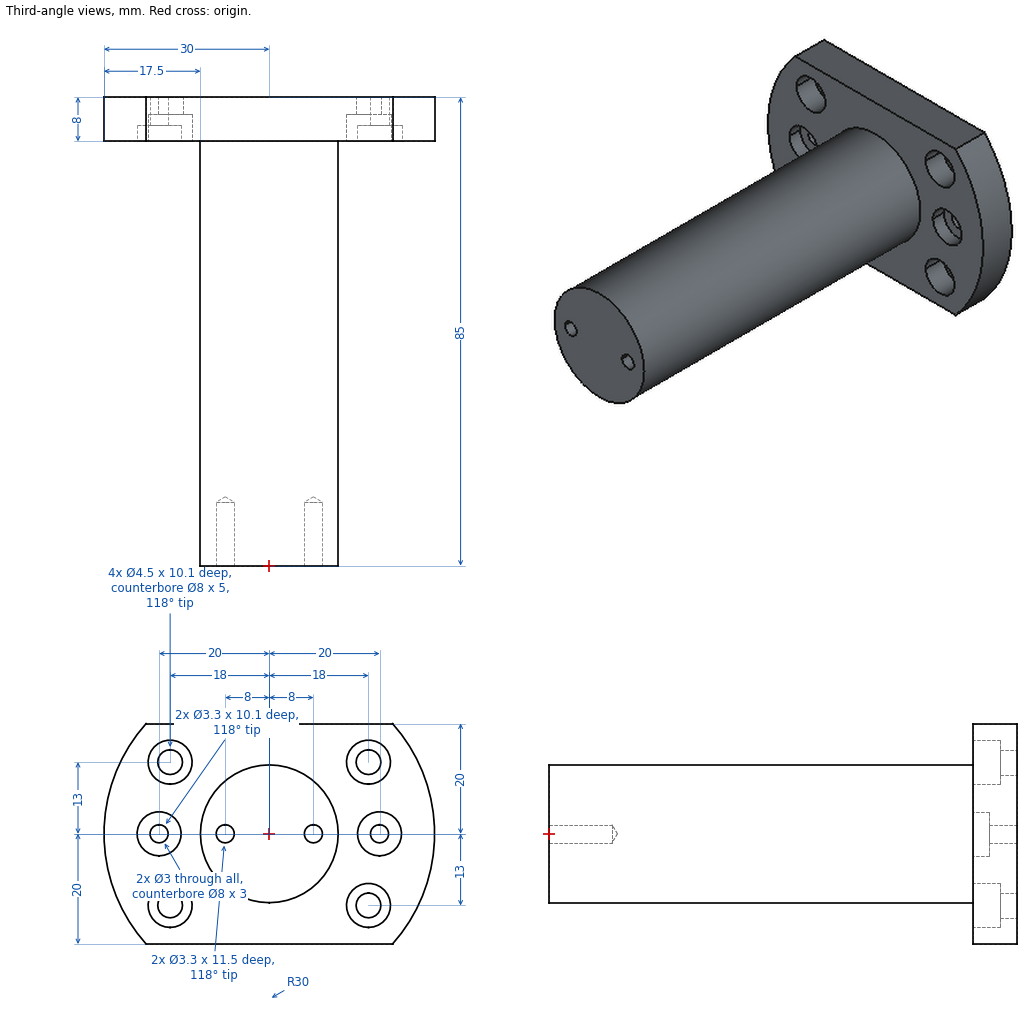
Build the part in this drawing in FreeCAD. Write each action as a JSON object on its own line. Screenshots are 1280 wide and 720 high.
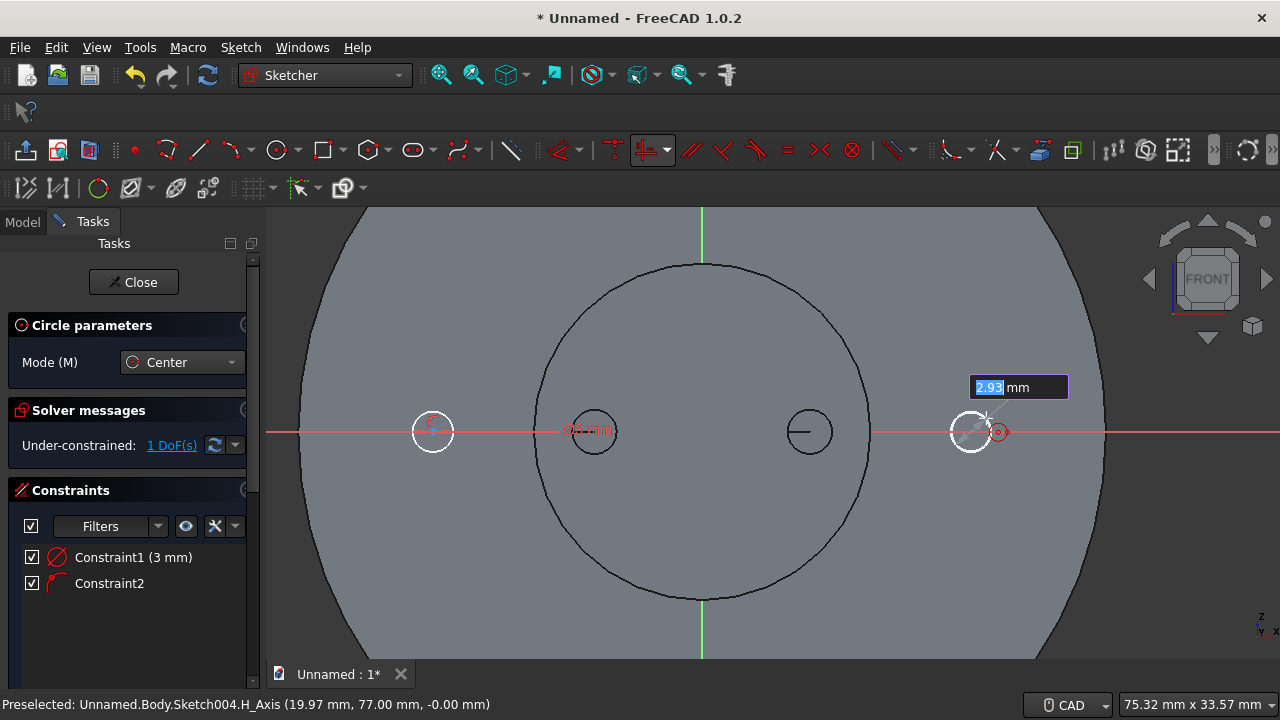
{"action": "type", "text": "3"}
{"action": "key", "text": "Return"}
{"action": "key", "text": "Escape"}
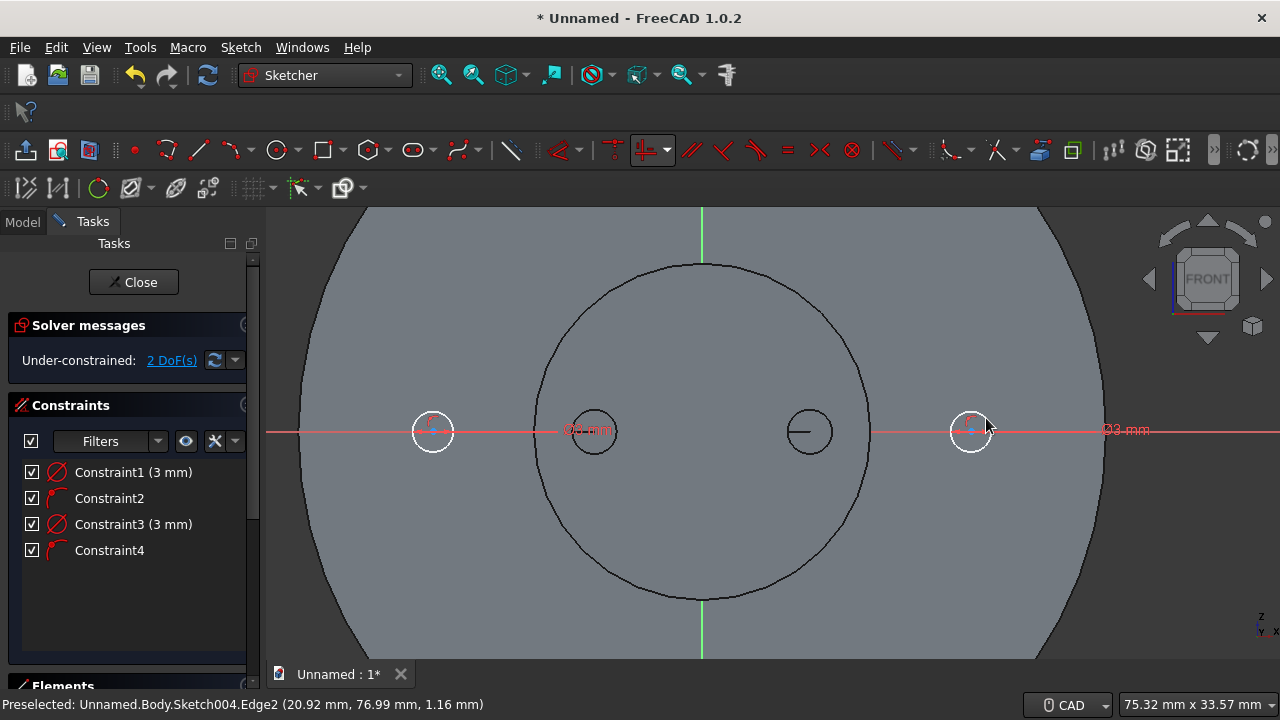
{"action": "left_click", "coordinate": [558, 150]}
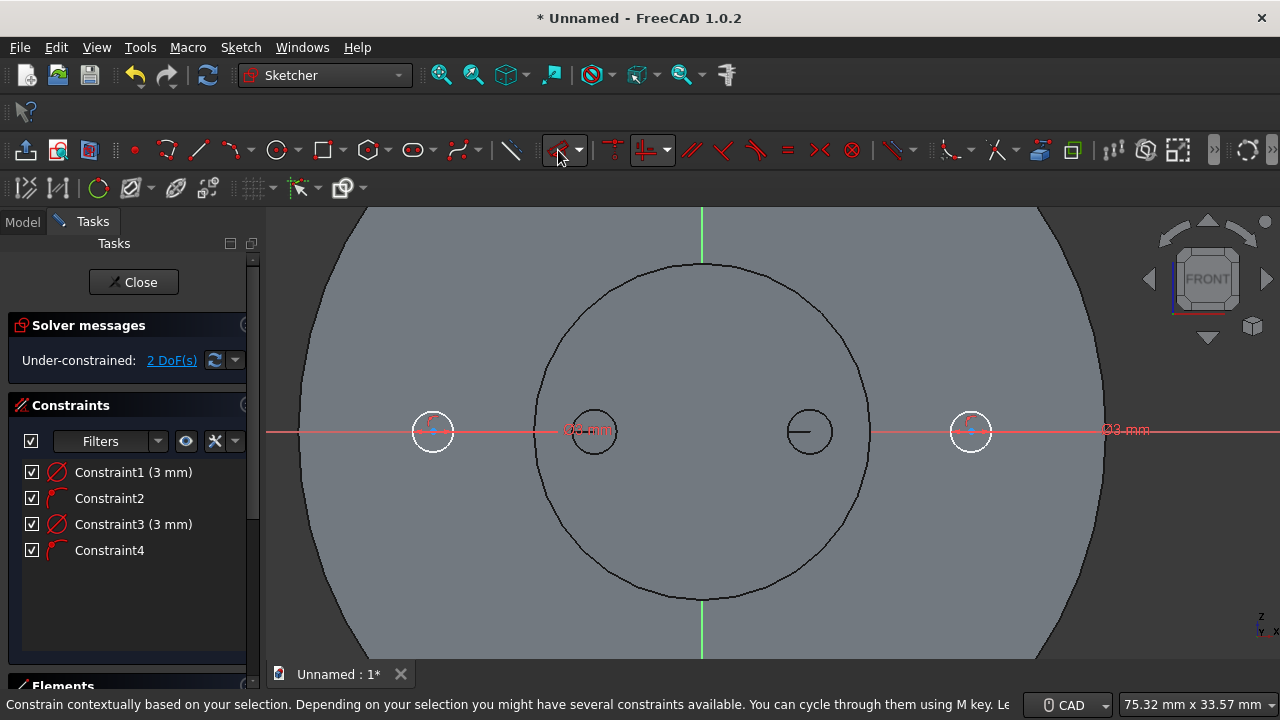
{"action": "left_click", "coordinate": [433, 432]}
{"action": "left_click", "coordinate": [568, 466]}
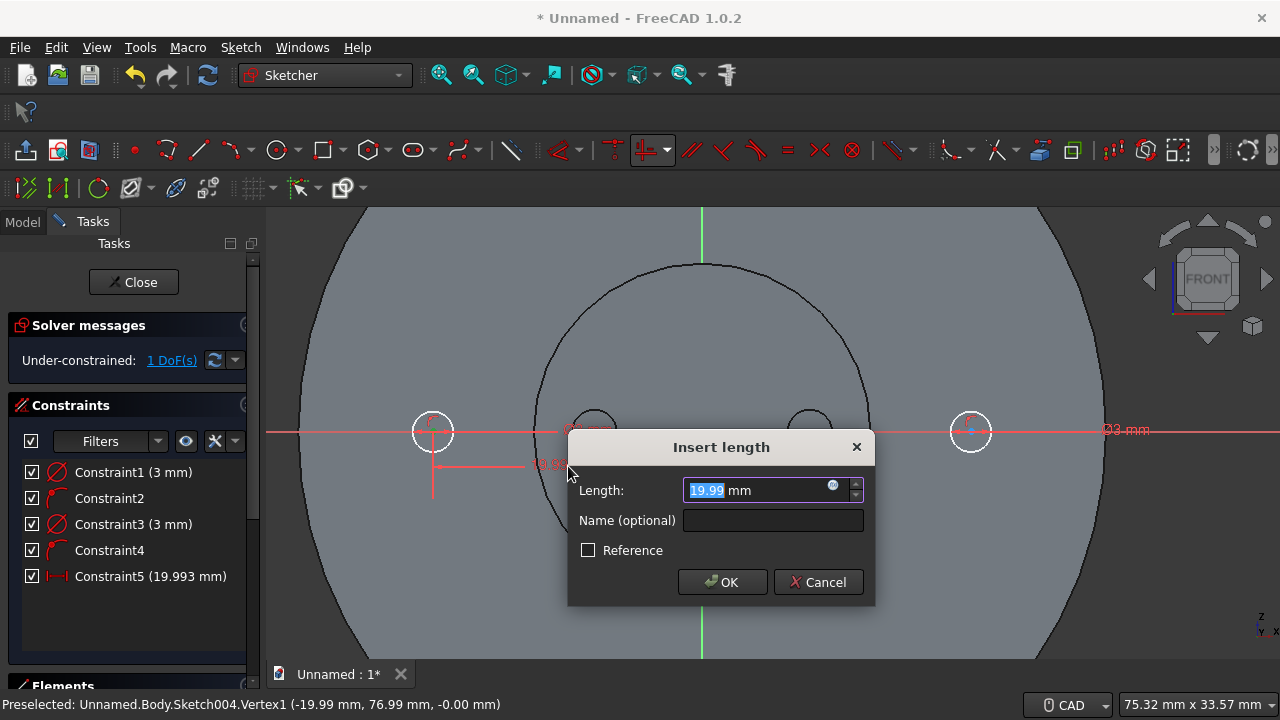
{"action": "type", "text": "20"}
{"action": "key", "text": "Return"}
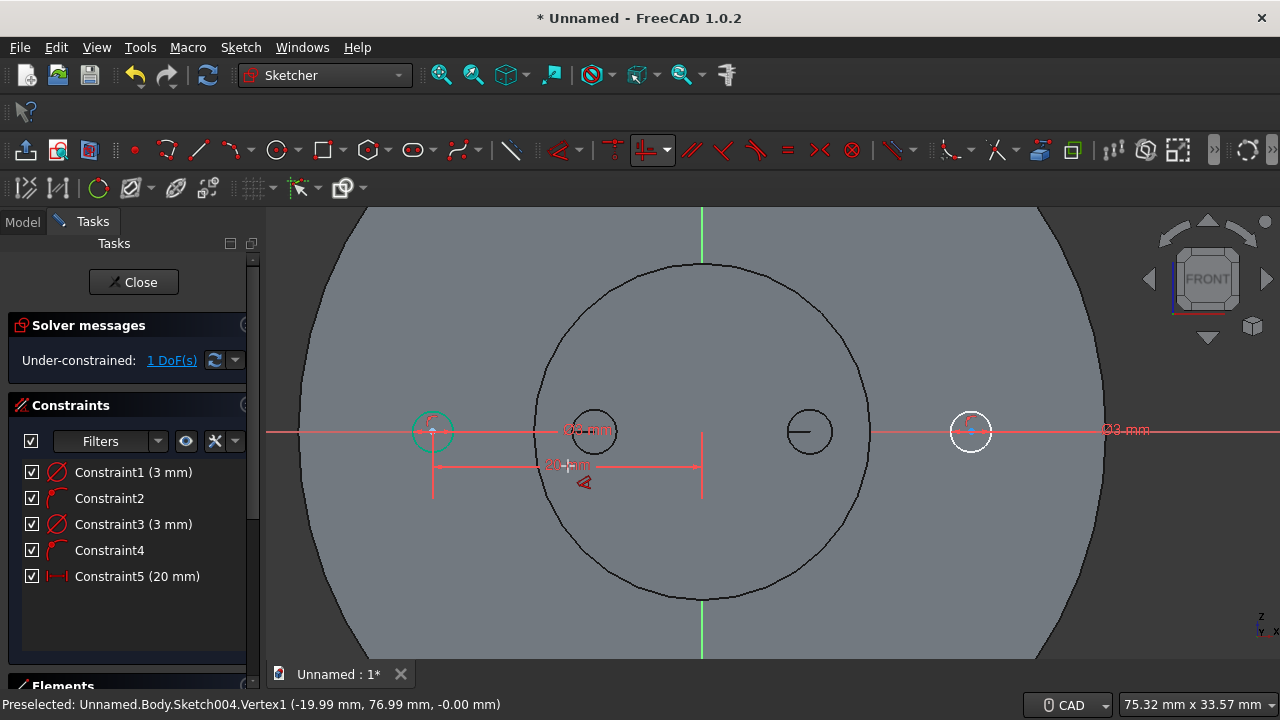
{"action": "left_click", "coordinate": [971, 432]}
{"action": "left_click", "coordinate": [837, 466]}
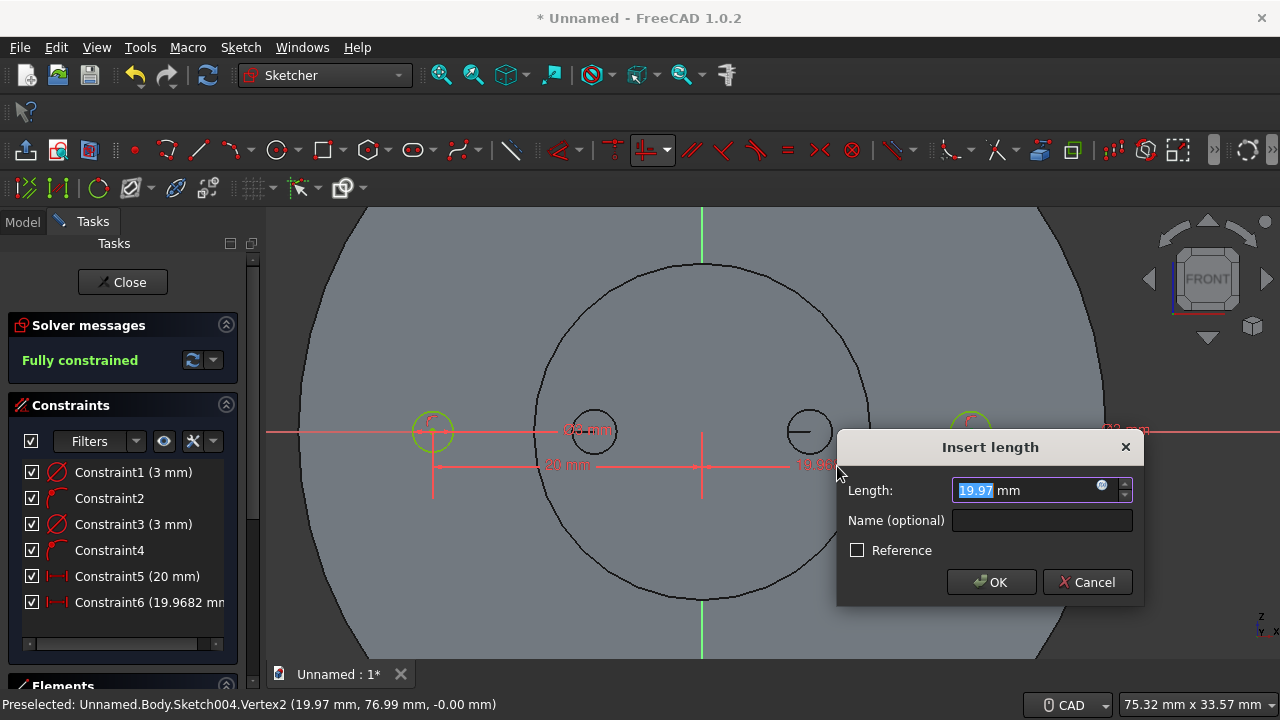
{"action": "type", "text": "20"}
{"action": "key", "text": "Return"}
{"action": "key", "text": "Escape"}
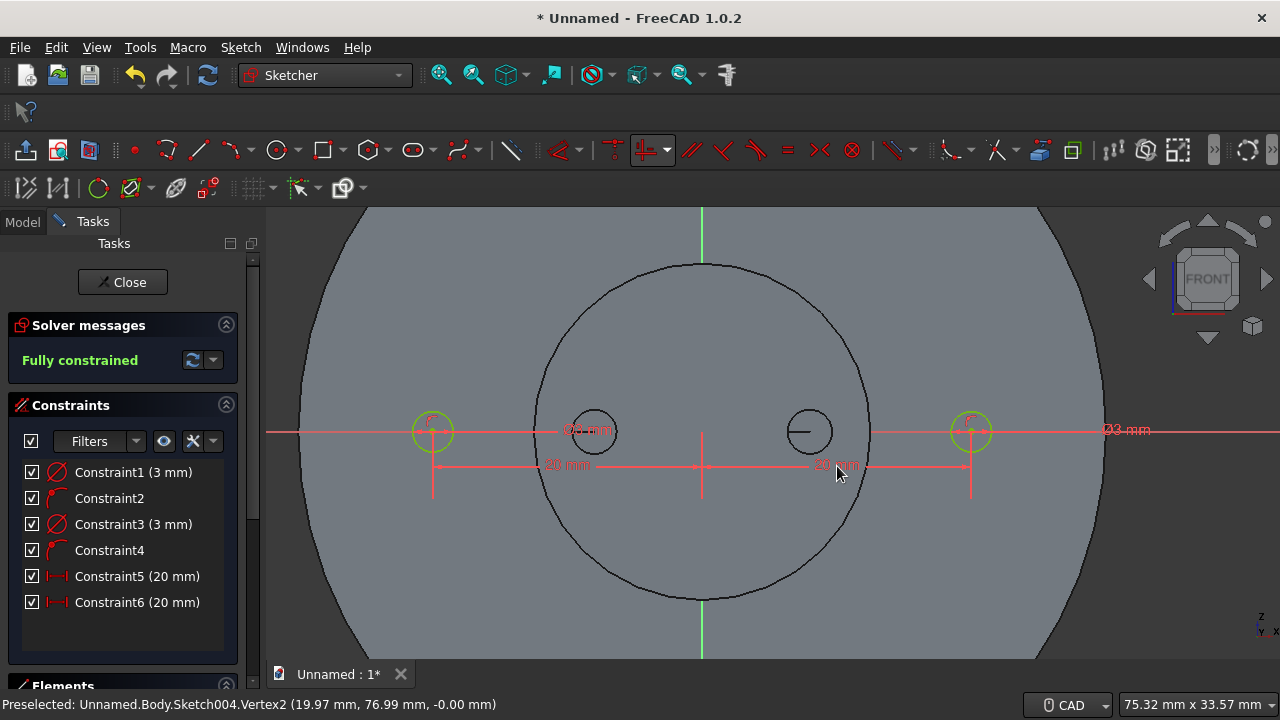
{"action": "left_click", "coordinate": [123, 282]}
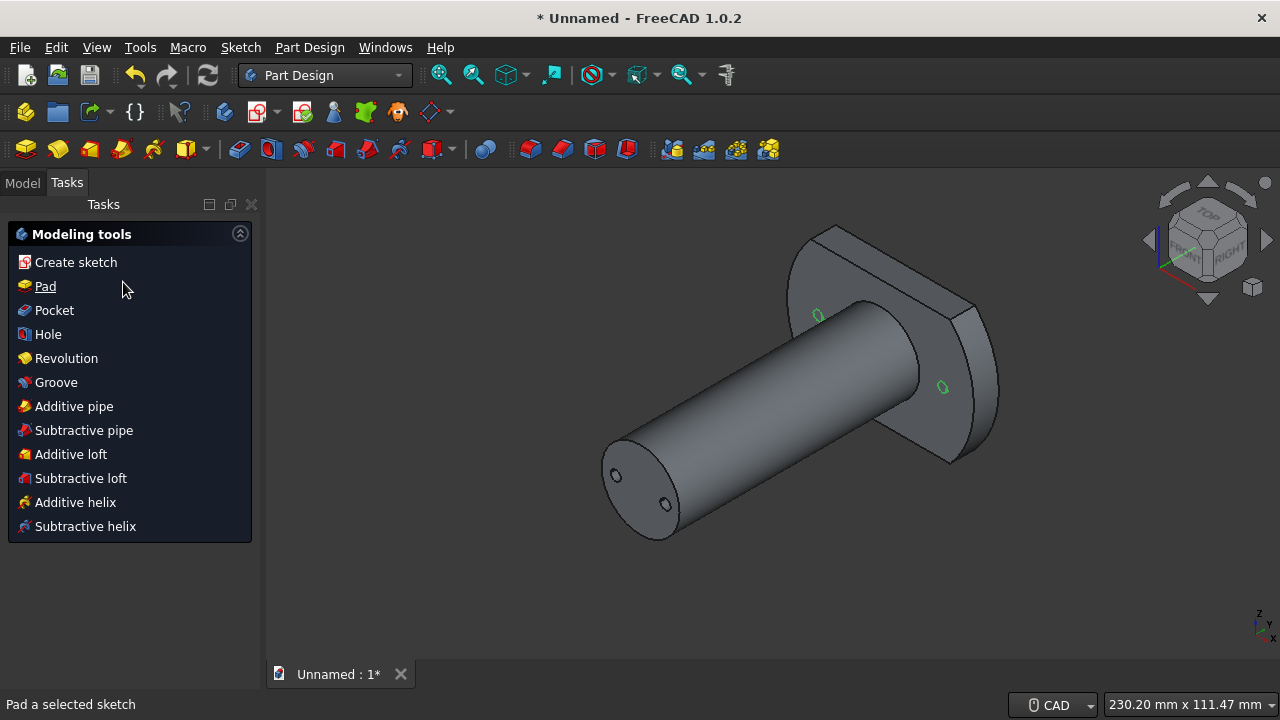
{"action": "left_click", "coordinate": [272, 150]}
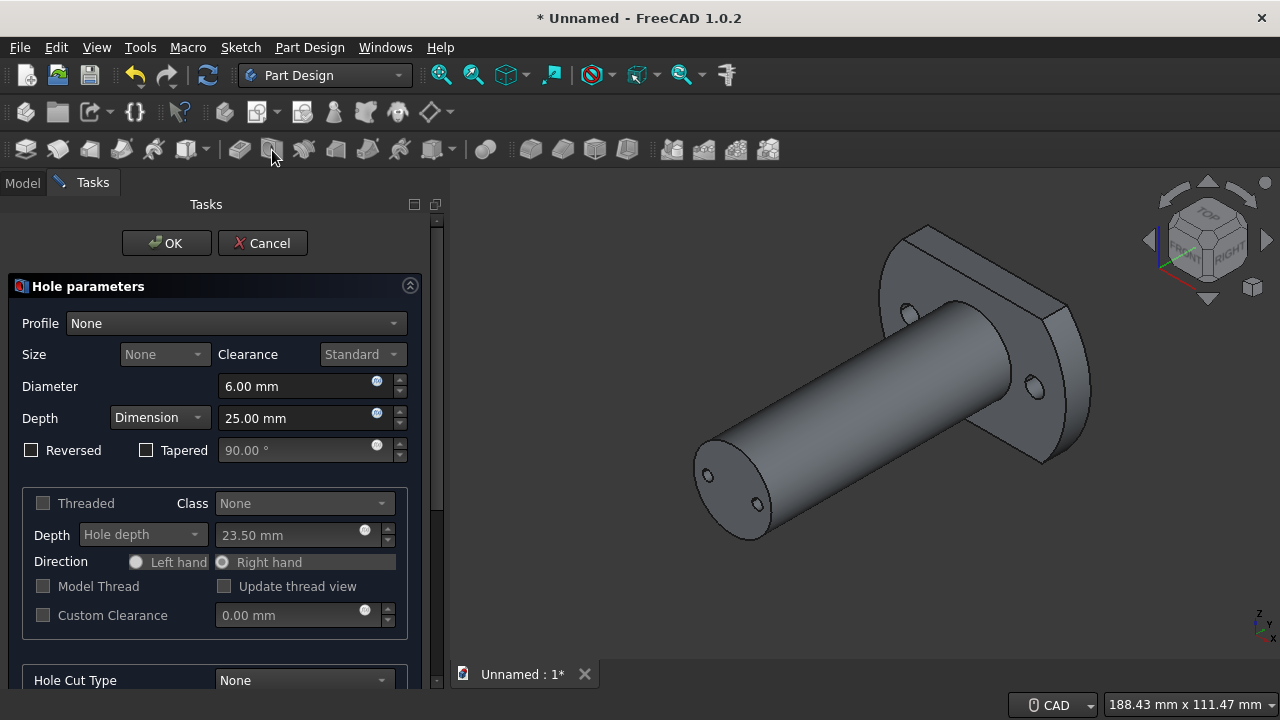
{"action": "triple_click", "coordinate": [305, 386]}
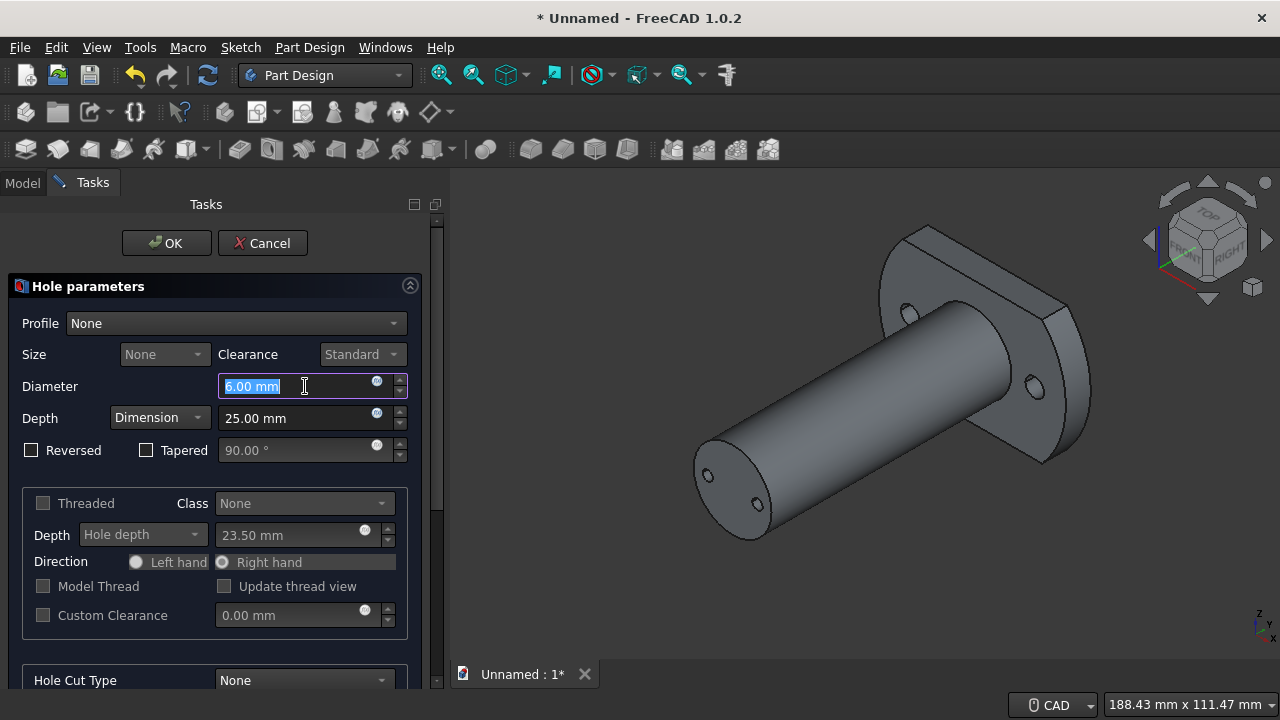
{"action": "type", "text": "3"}
{"action": "key", "text": "Tab"}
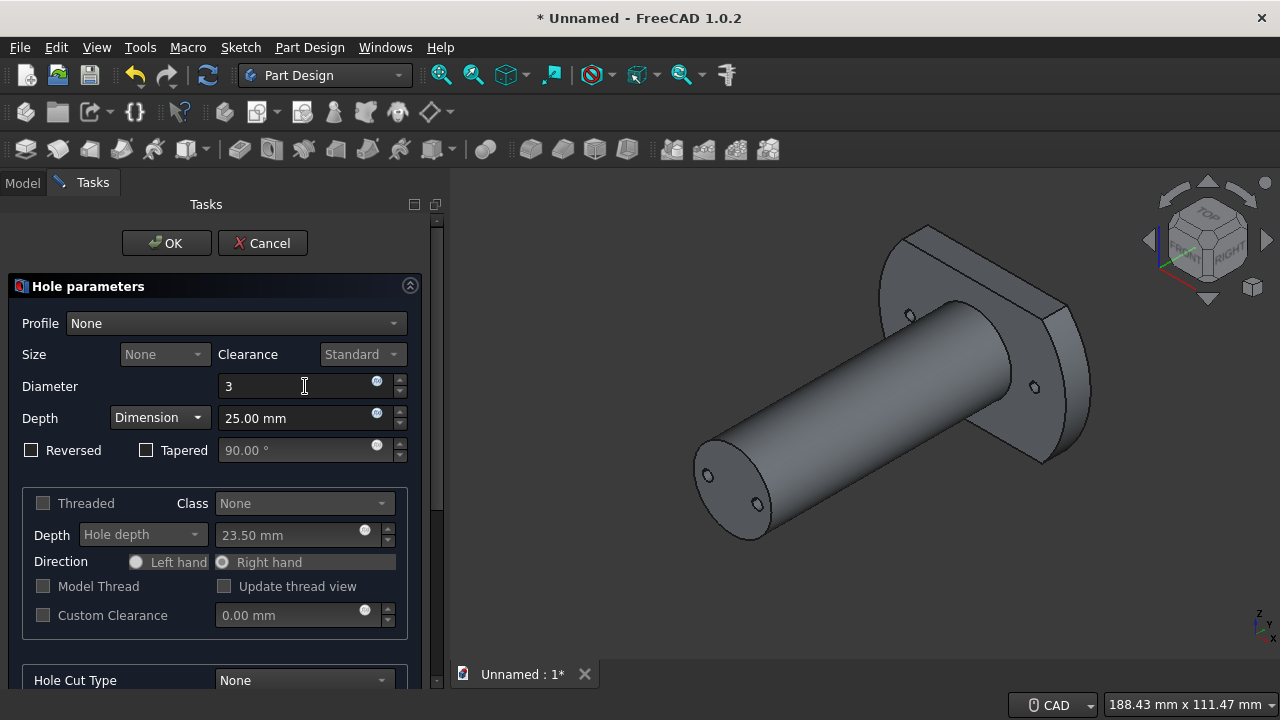
{"action": "left_click", "coordinate": [161, 418]}